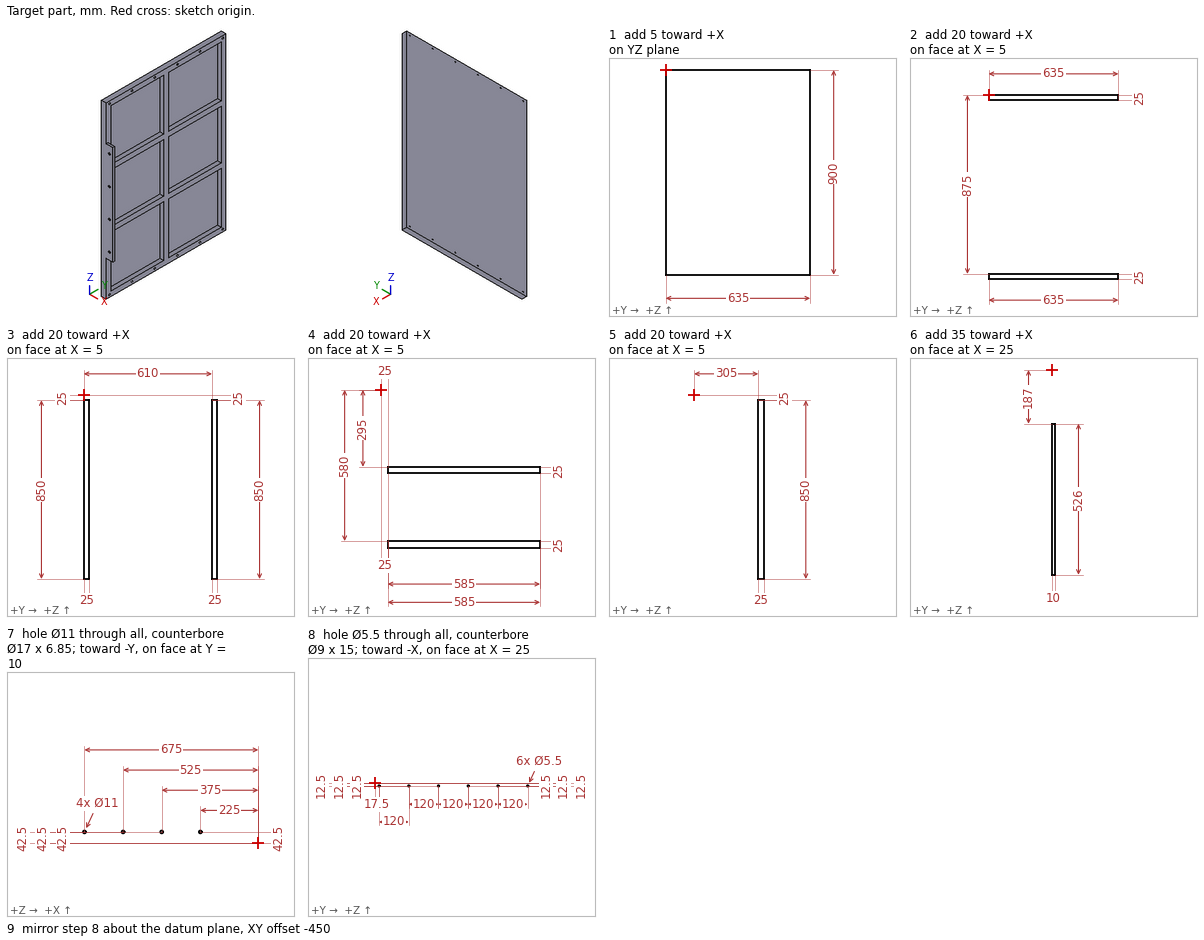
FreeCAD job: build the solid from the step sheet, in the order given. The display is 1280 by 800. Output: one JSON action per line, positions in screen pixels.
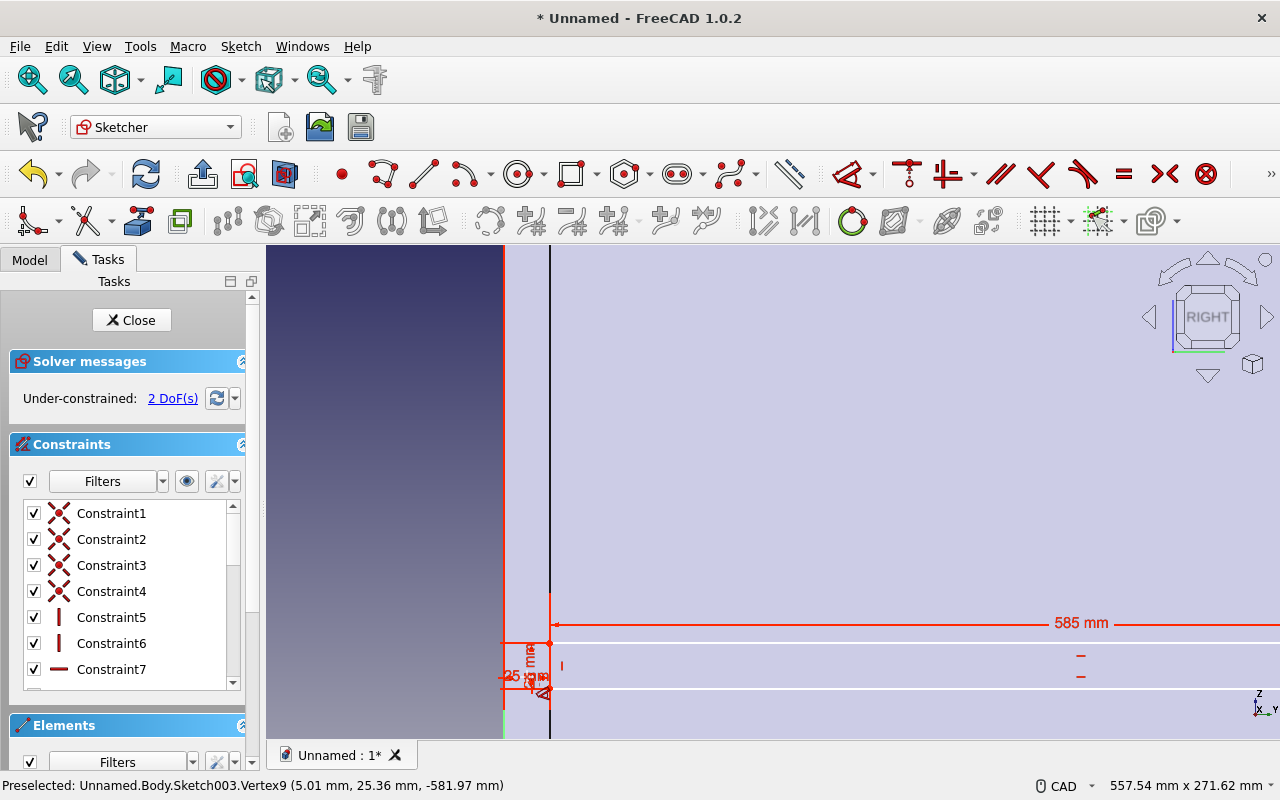
{"action": "scroll", "coordinate": [552, 646], "scroll_direction": "down", "scroll_amount": 6}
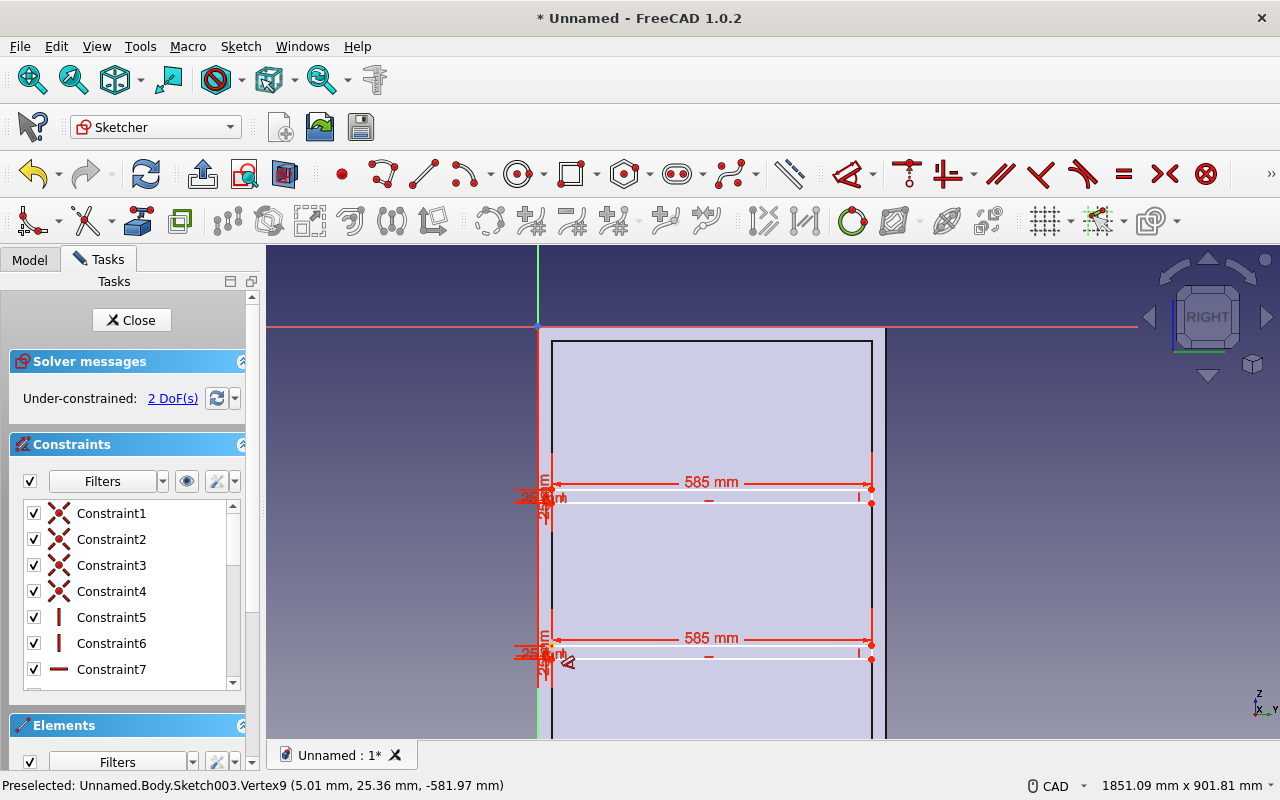
{"action": "left_click", "coordinate": [552, 490]}
{"action": "left_click", "coordinate": [504, 408]}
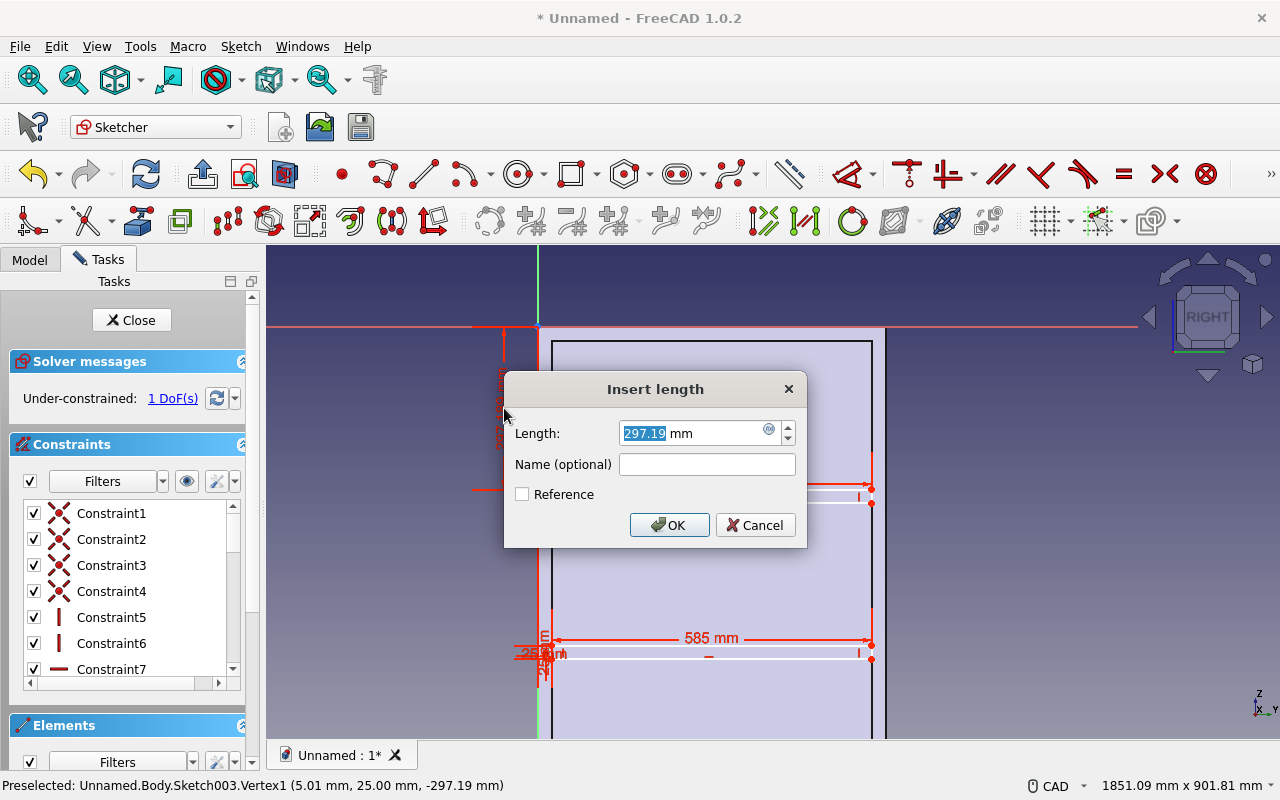
{"action": "type", "text": "295"}
{"action": "key", "text": "Return"}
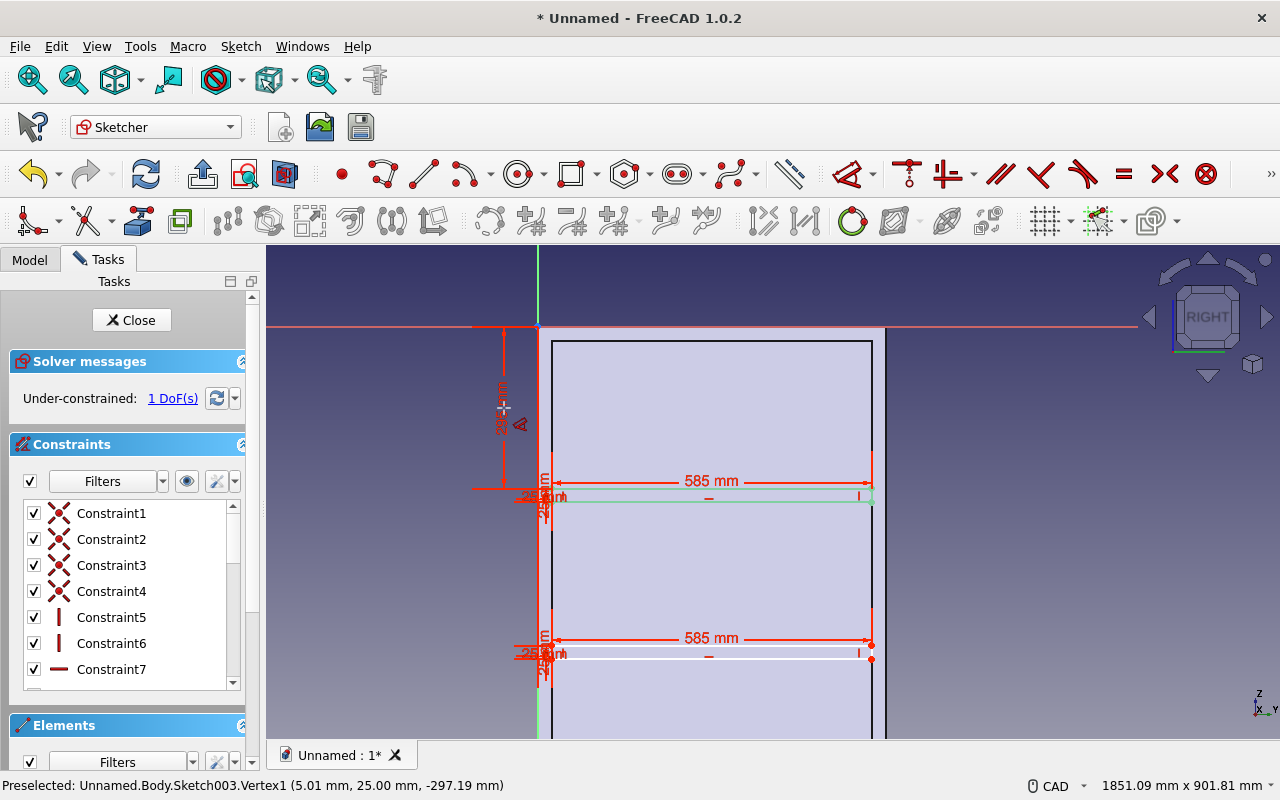
{"action": "left_click", "coordinate": [552, 646]}
{"action": "left_click", "coordinate": [504, 560]}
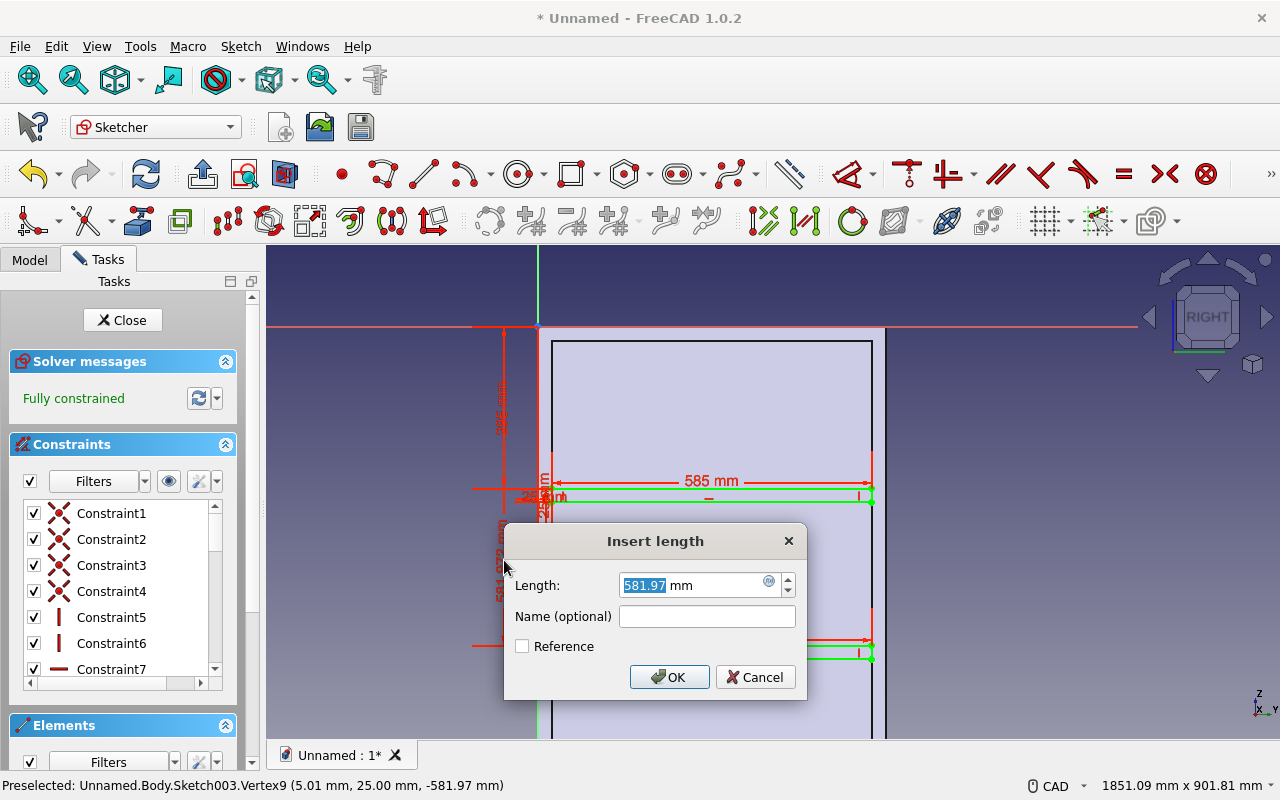
{"action": "type", "text": "580"}
{"action": "key", "text": "Return"}
{"action": "key", "text": "Escape"}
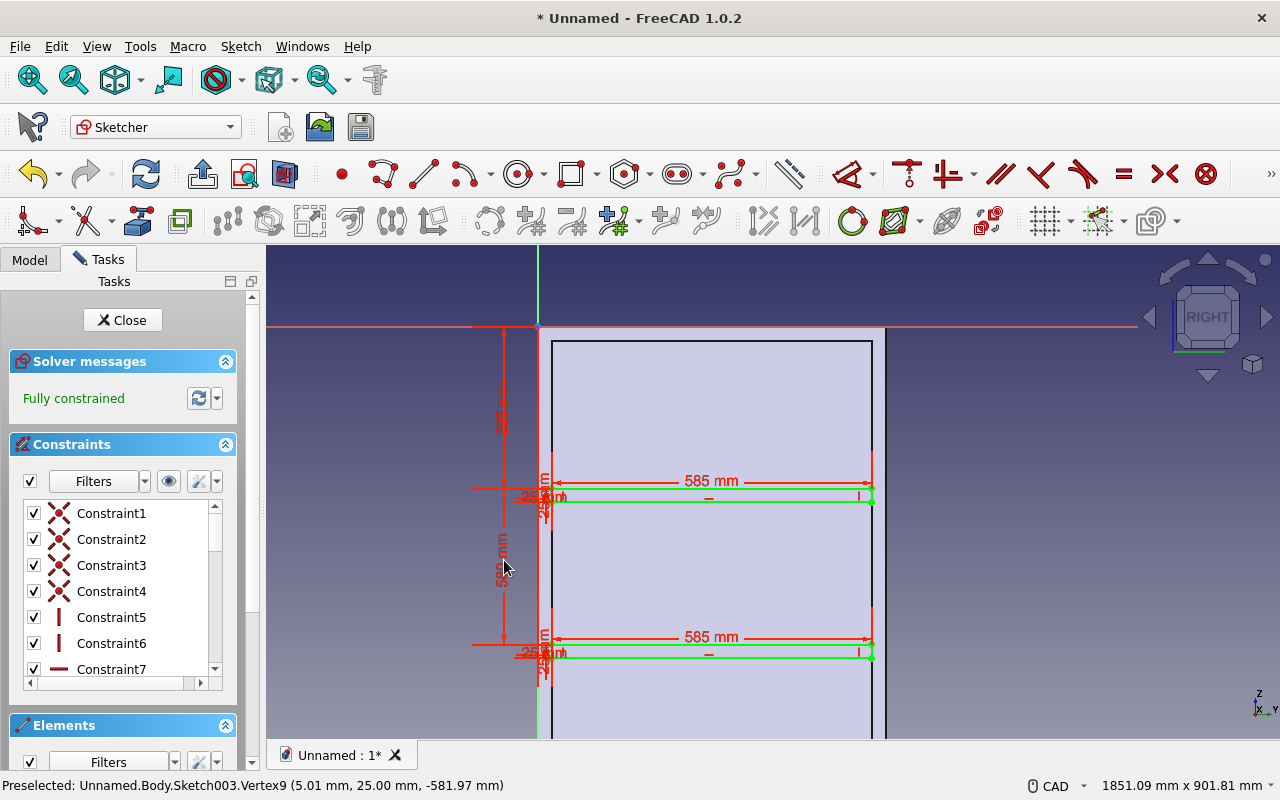
{"action": "left_click", "coordinate": [123, 320]}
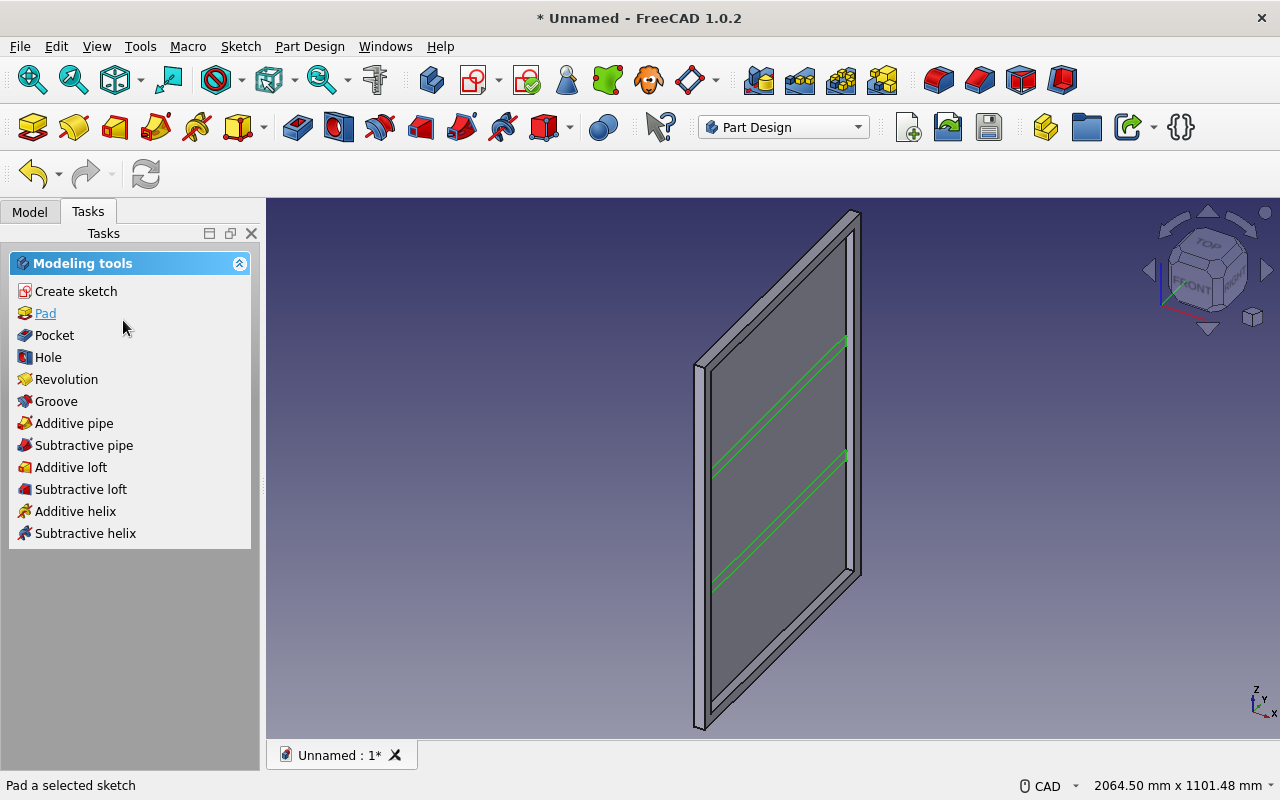
{"action": "left_click", "coordinate": [33, 128]}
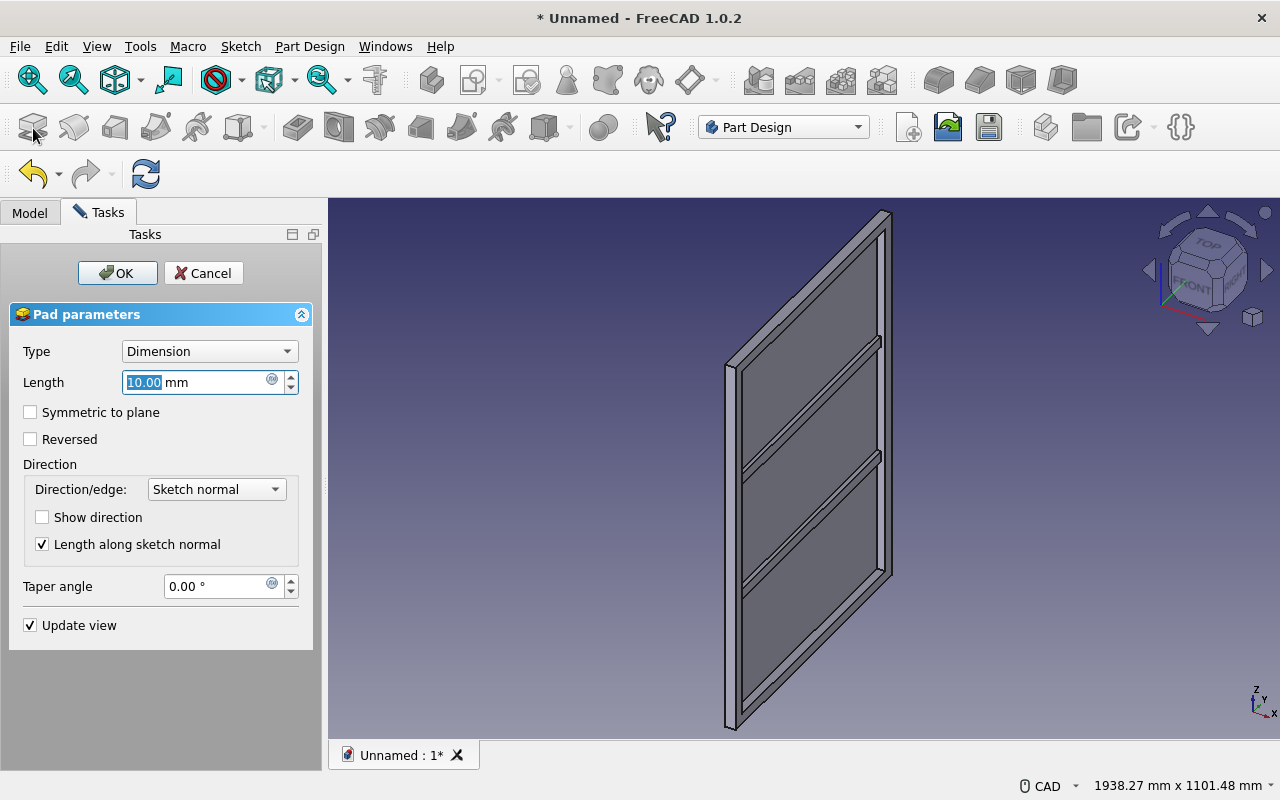
{"action": "type", "text": "20"}
{"action": "key", "text": "Tab"}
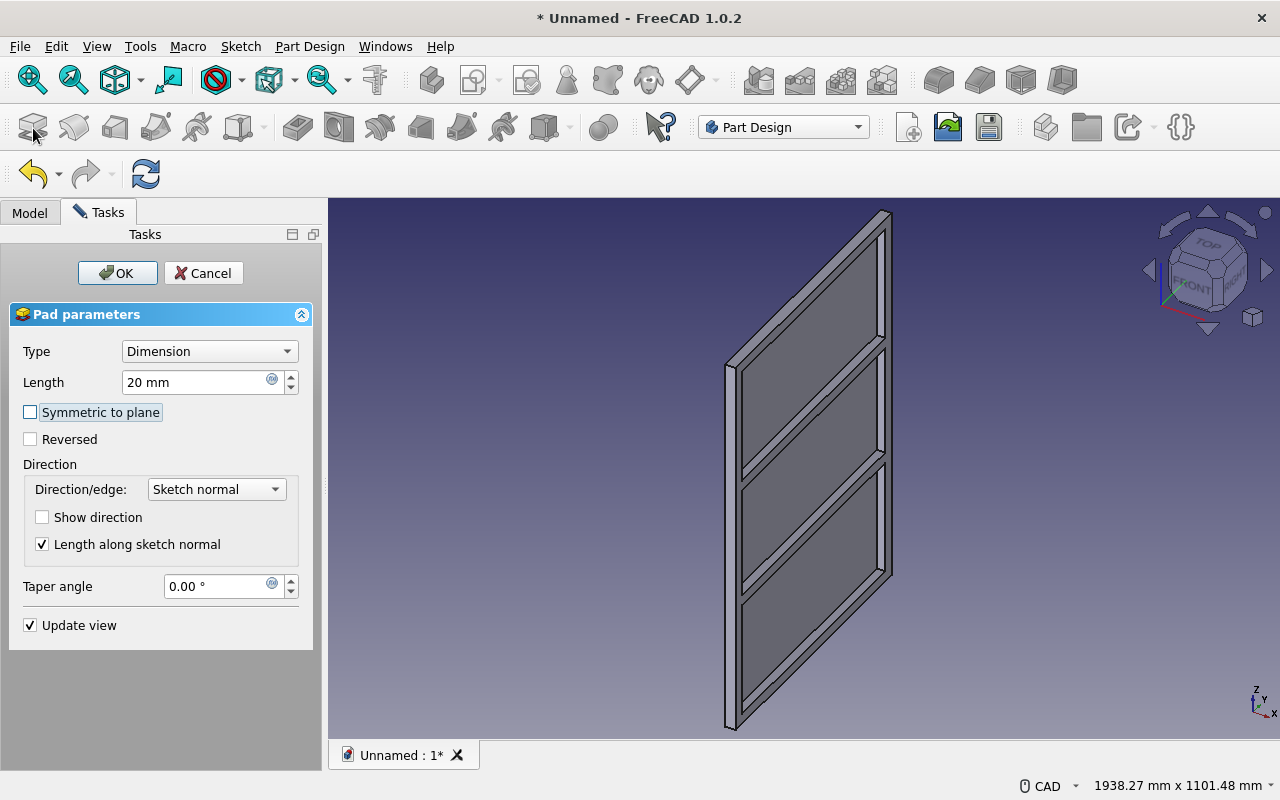
{"action": "left_click", "coordinate": [118, 273]}